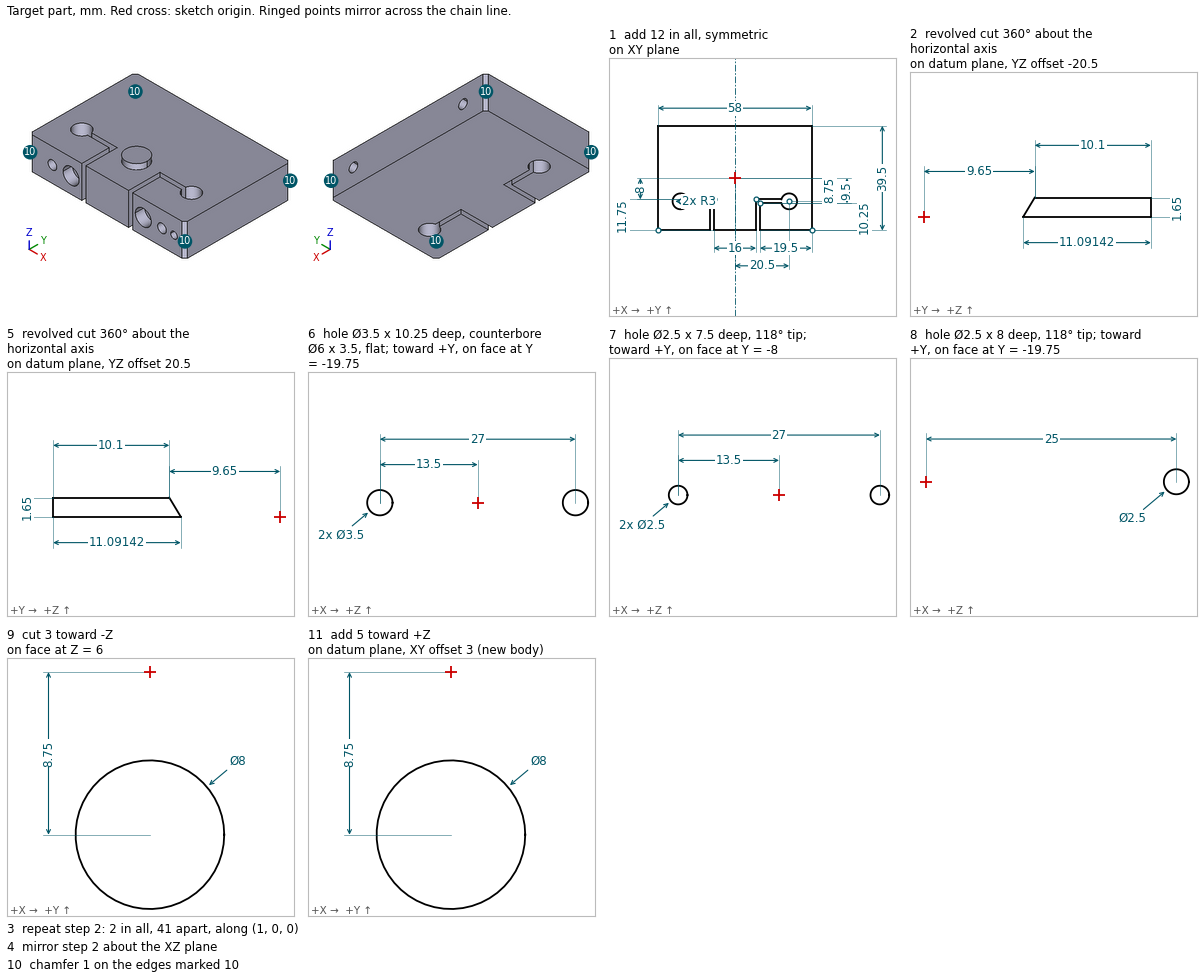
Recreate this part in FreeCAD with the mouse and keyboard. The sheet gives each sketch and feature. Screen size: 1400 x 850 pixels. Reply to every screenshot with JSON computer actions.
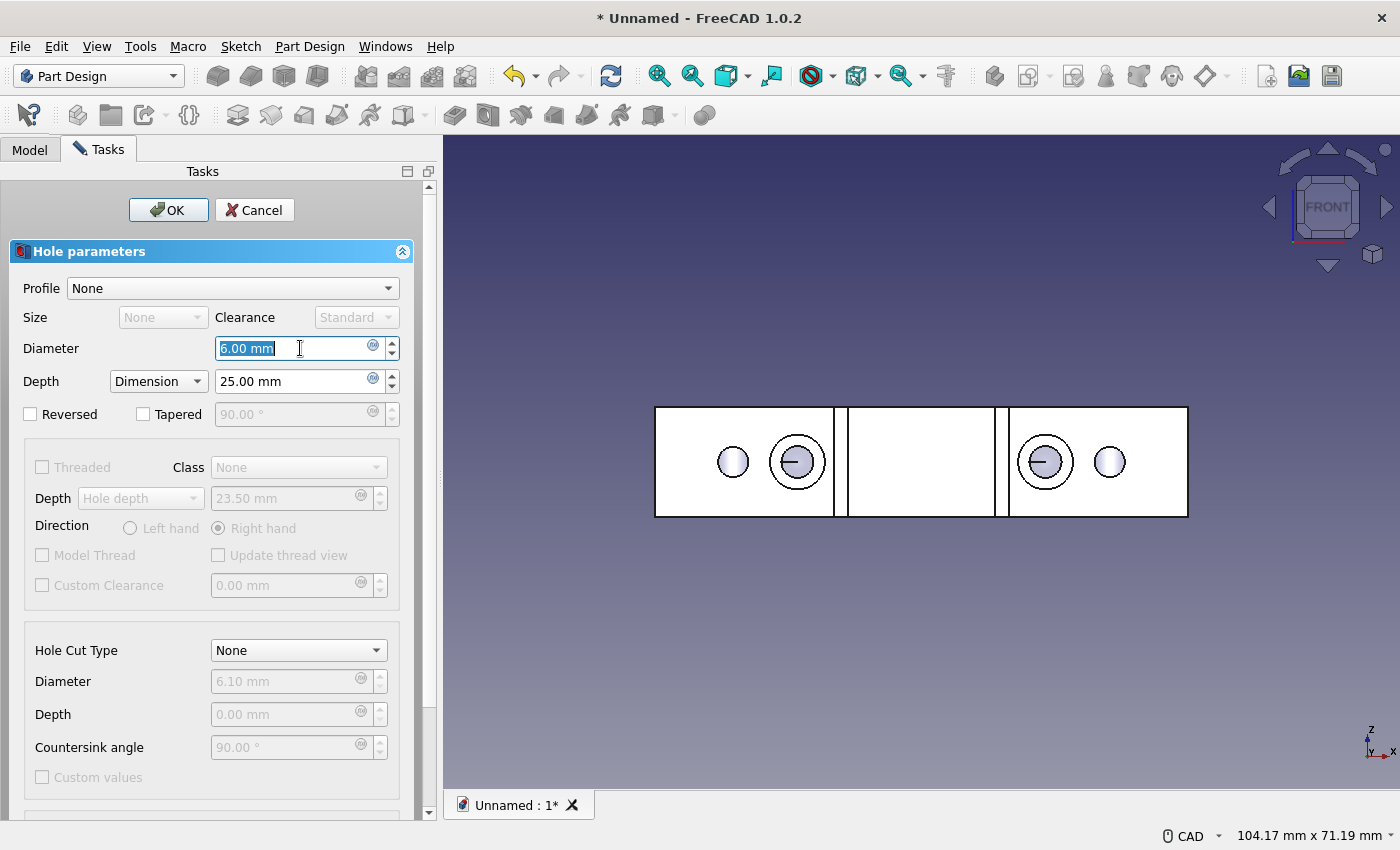
{"action": "type", "text": "2.5"}
{"action": "key", "text": "Tab"}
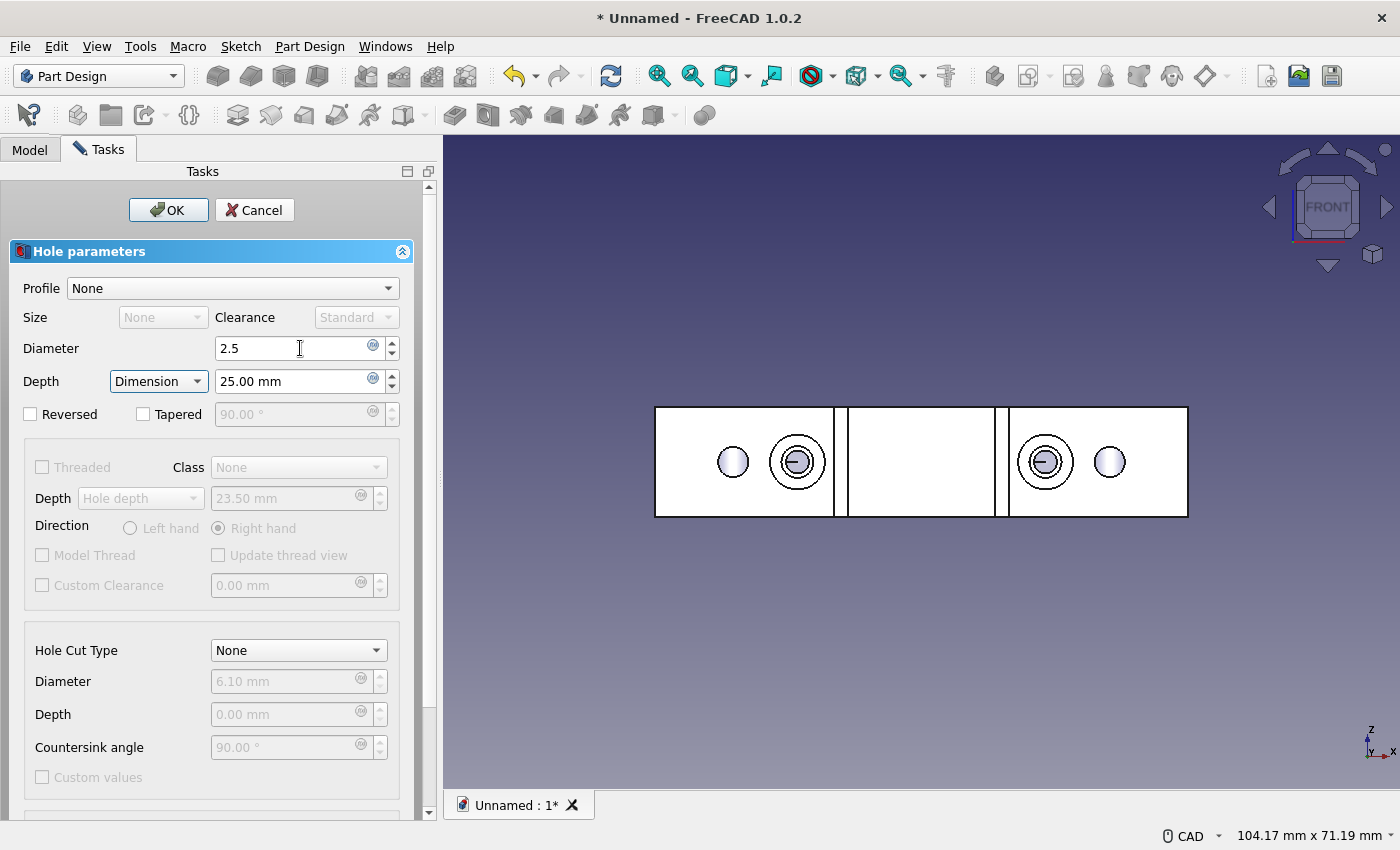
{"action": "triple_click", "coordinate": [300, 382]}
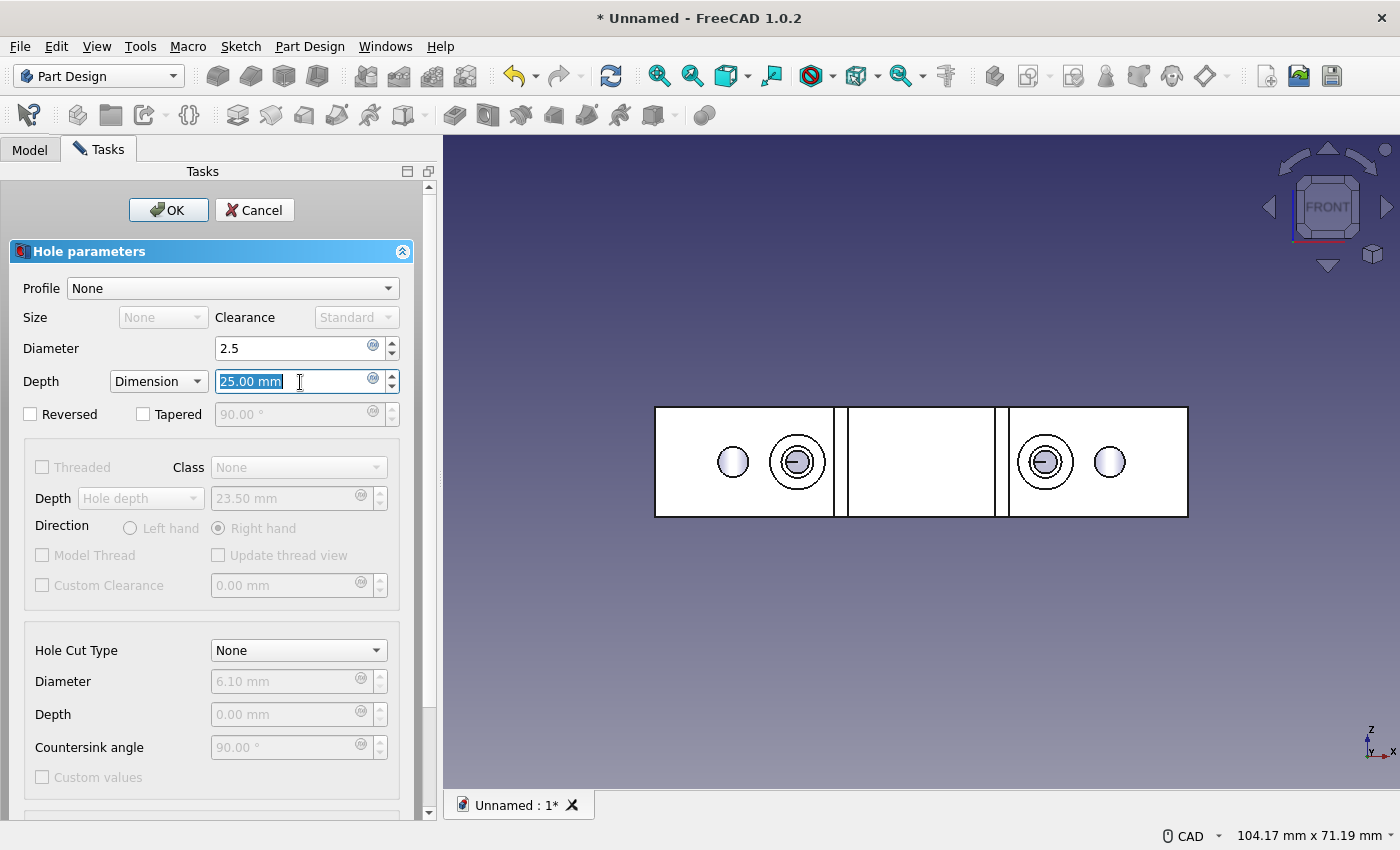
{"action": "type", "text": "7.5"}
{"action": "key", "text": "Tab"}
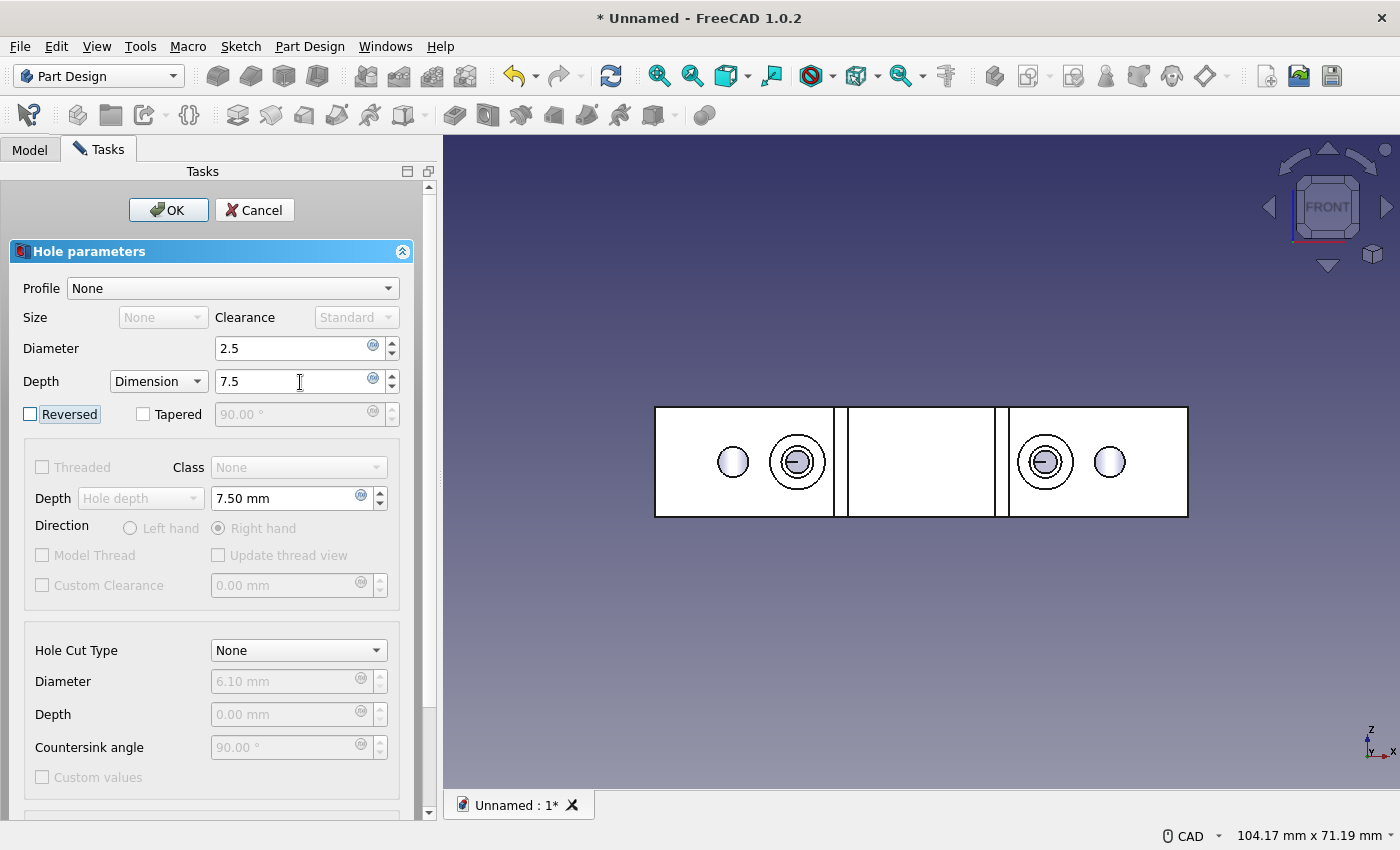
{"action": "left_click", "coordinate": [169, 210]}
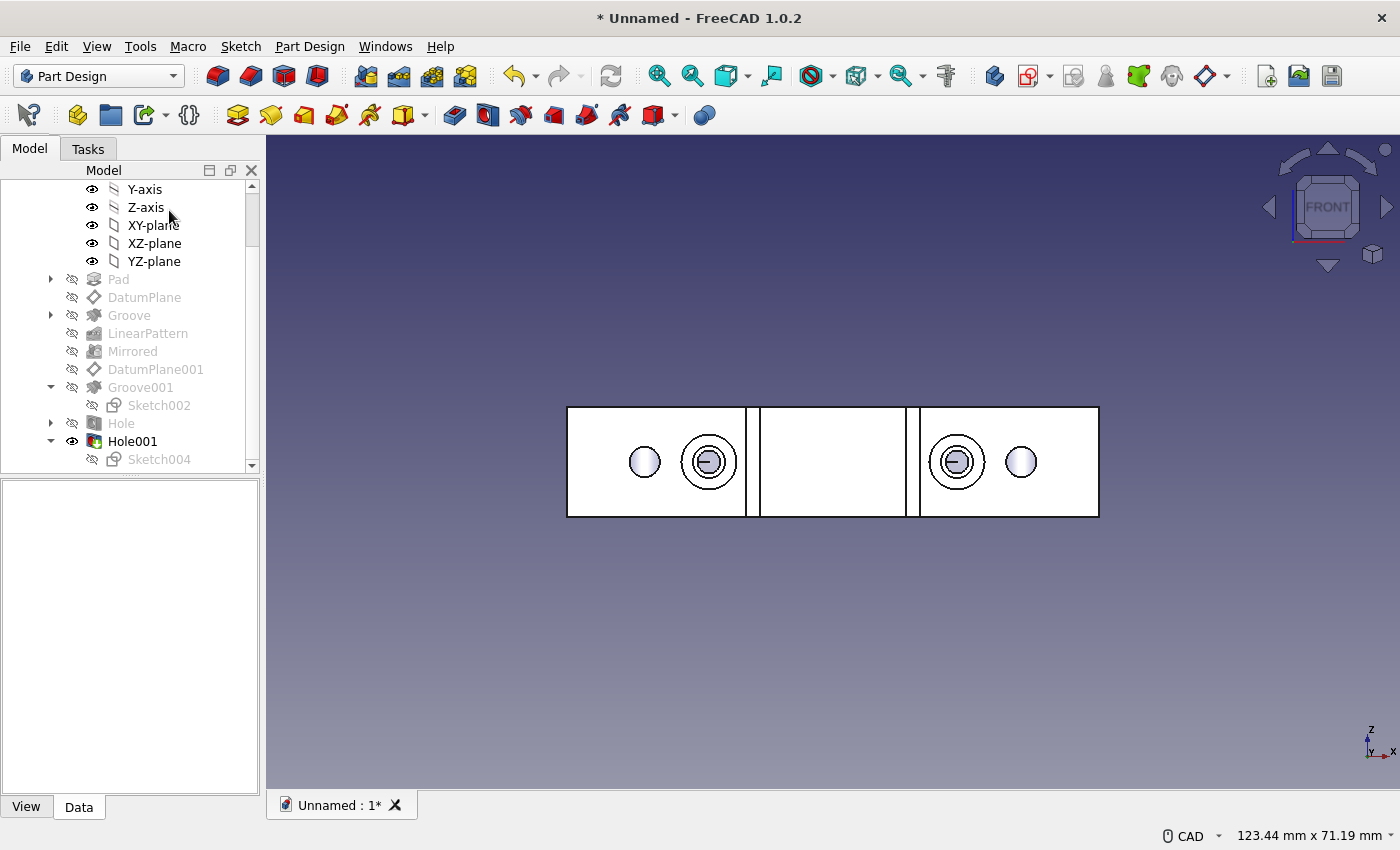
{"action": "left_click", "coordinate": [605, 445]}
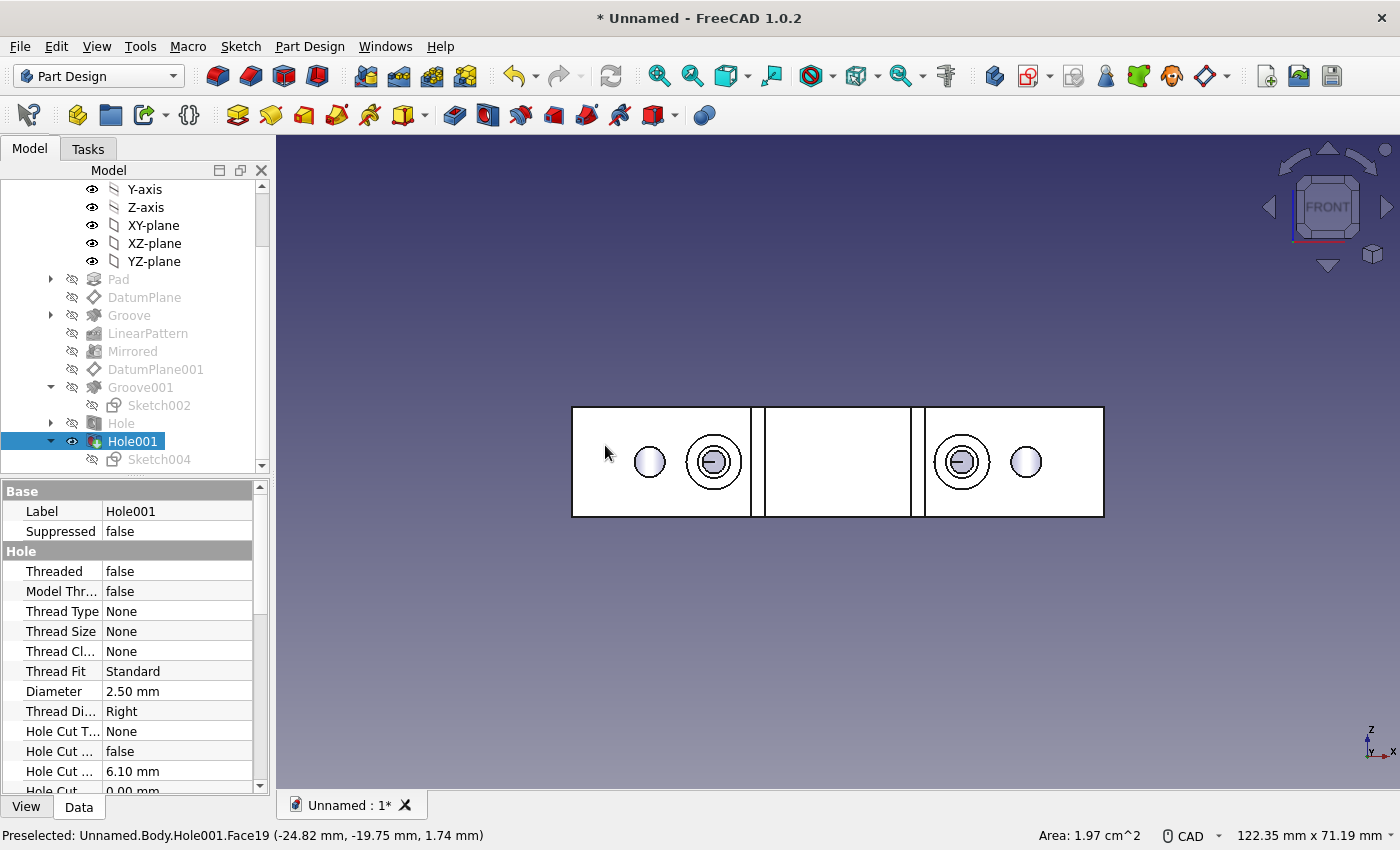
{"action": "left_click", "coordinate": [1028, 76]}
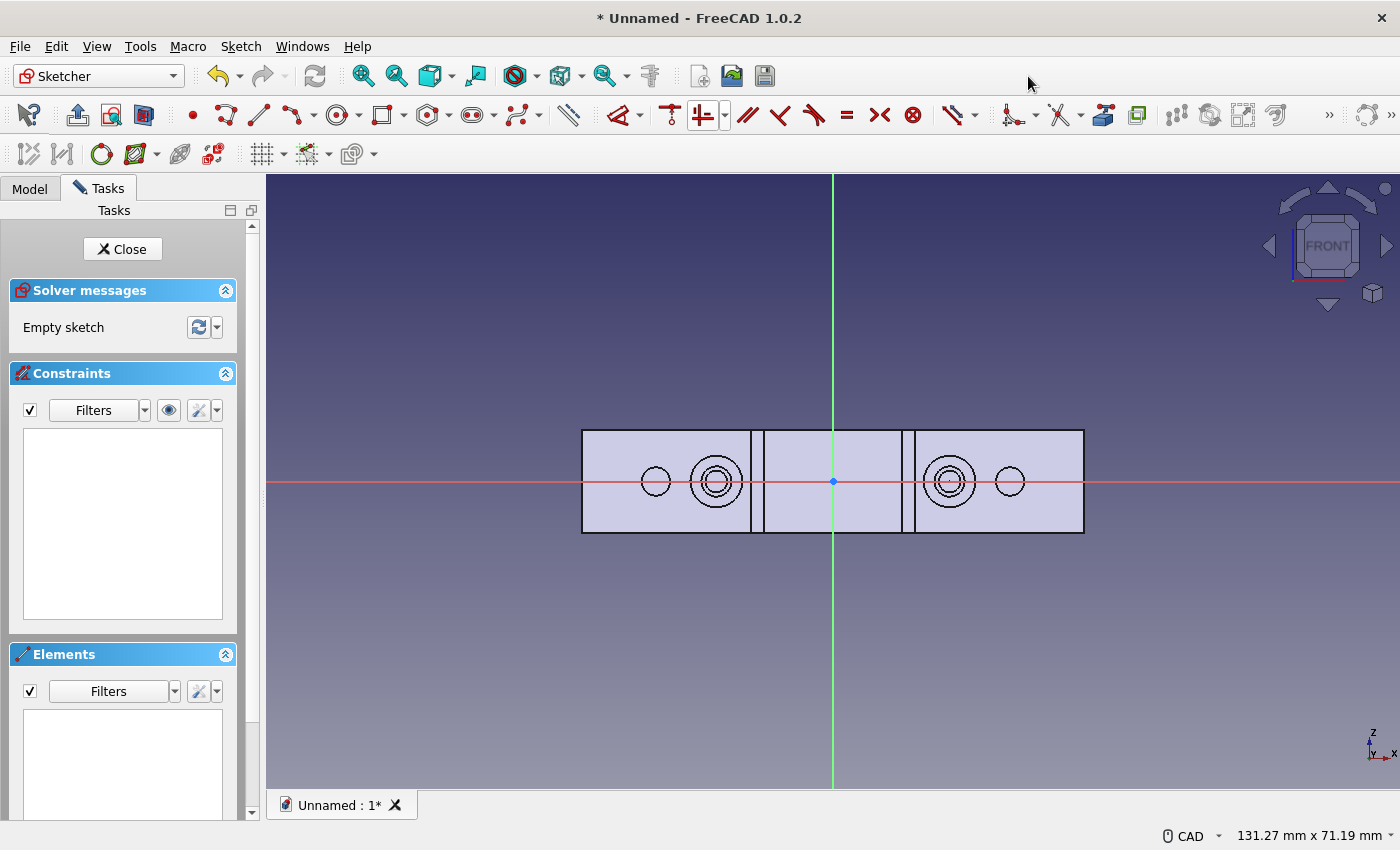
{"action": "scroll", "coordinate": [1064, 482], "scroll_direction": "up", "scroll_amount": 15}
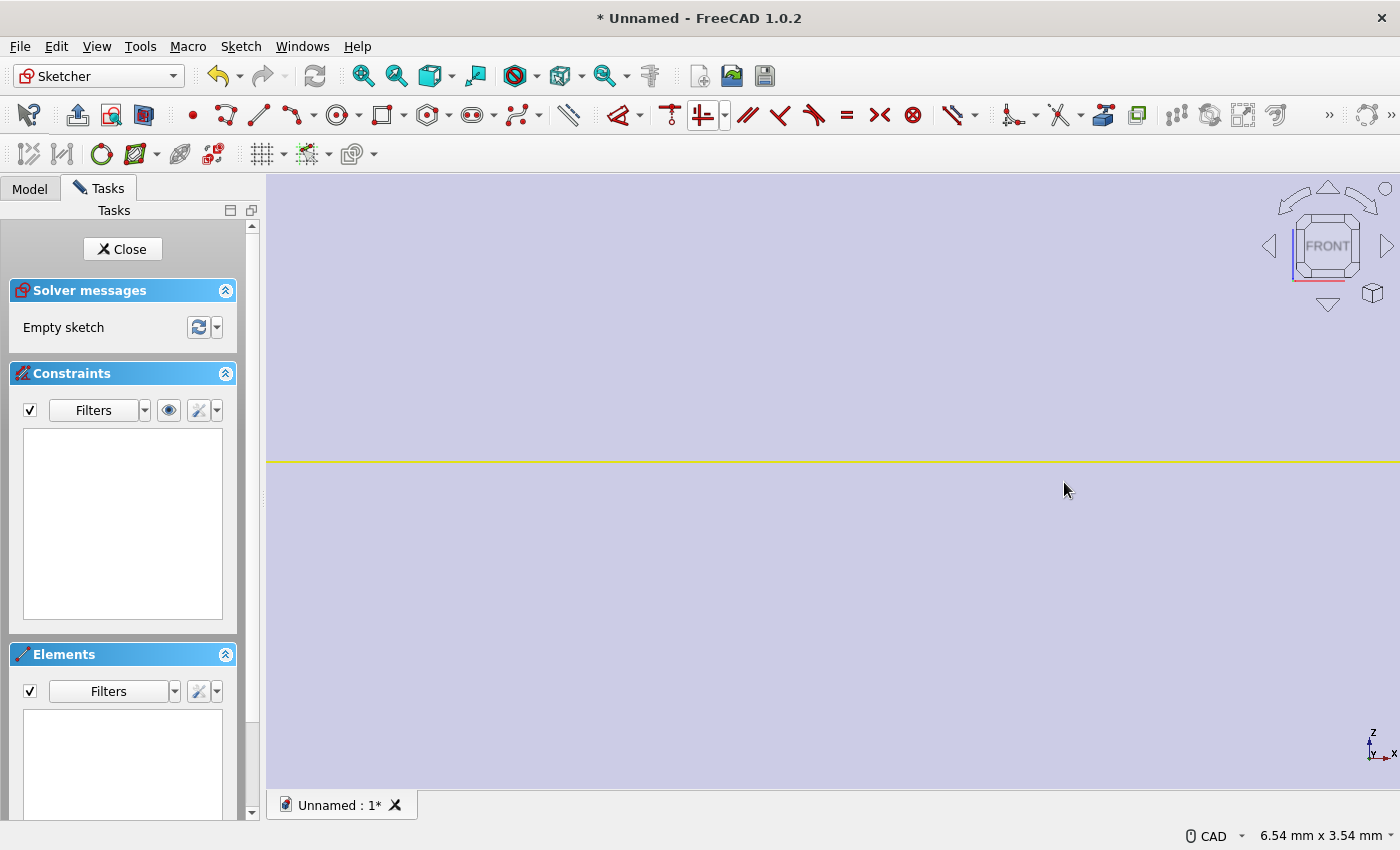
{"action": "left_click", "coordinate": [336, 116]}